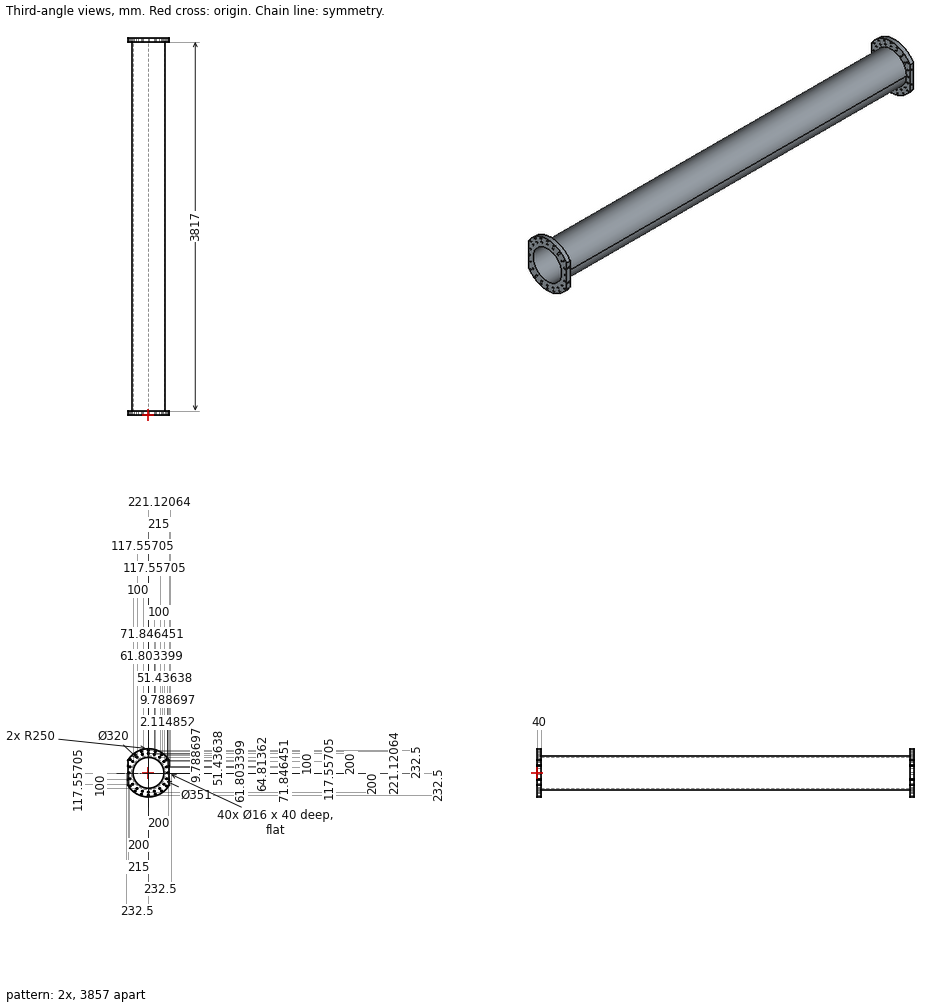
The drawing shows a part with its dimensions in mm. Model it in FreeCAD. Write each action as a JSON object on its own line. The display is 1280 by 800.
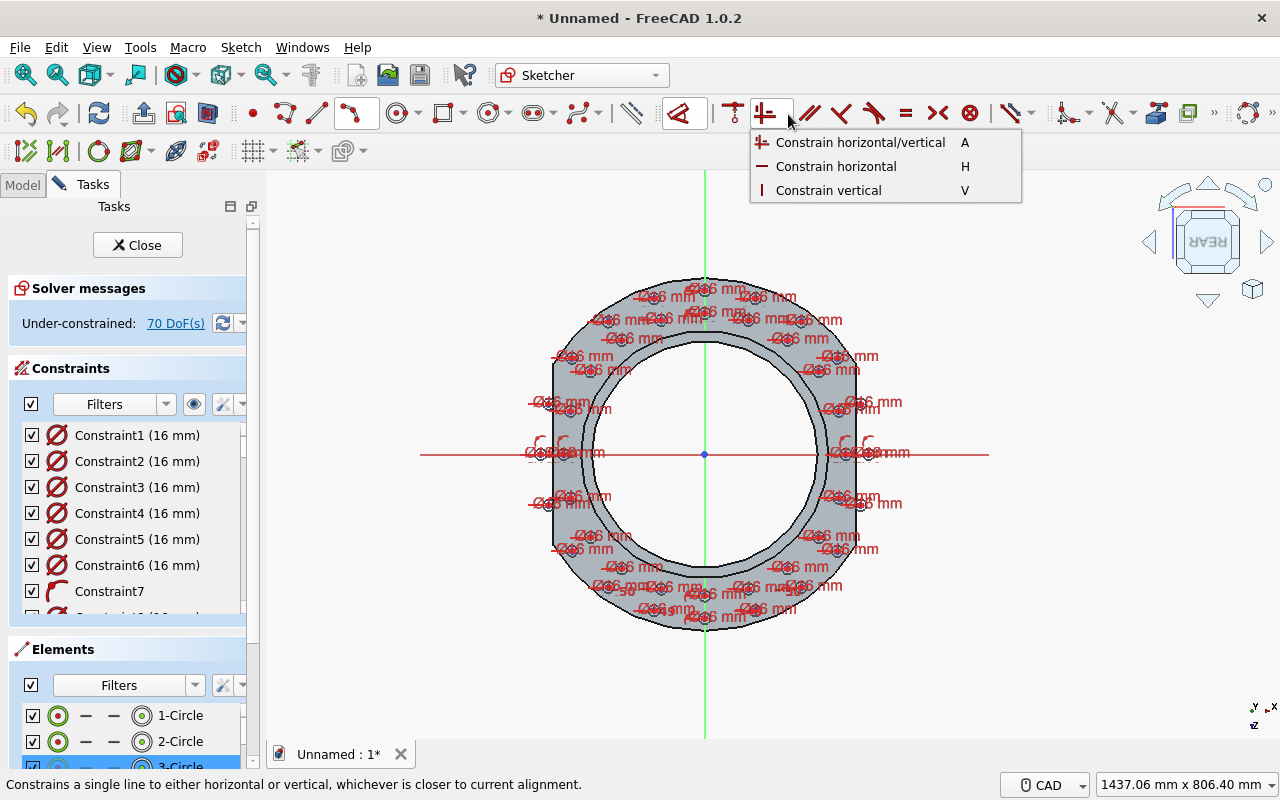
{"action": "left_click", "coordinate": [886, 166]}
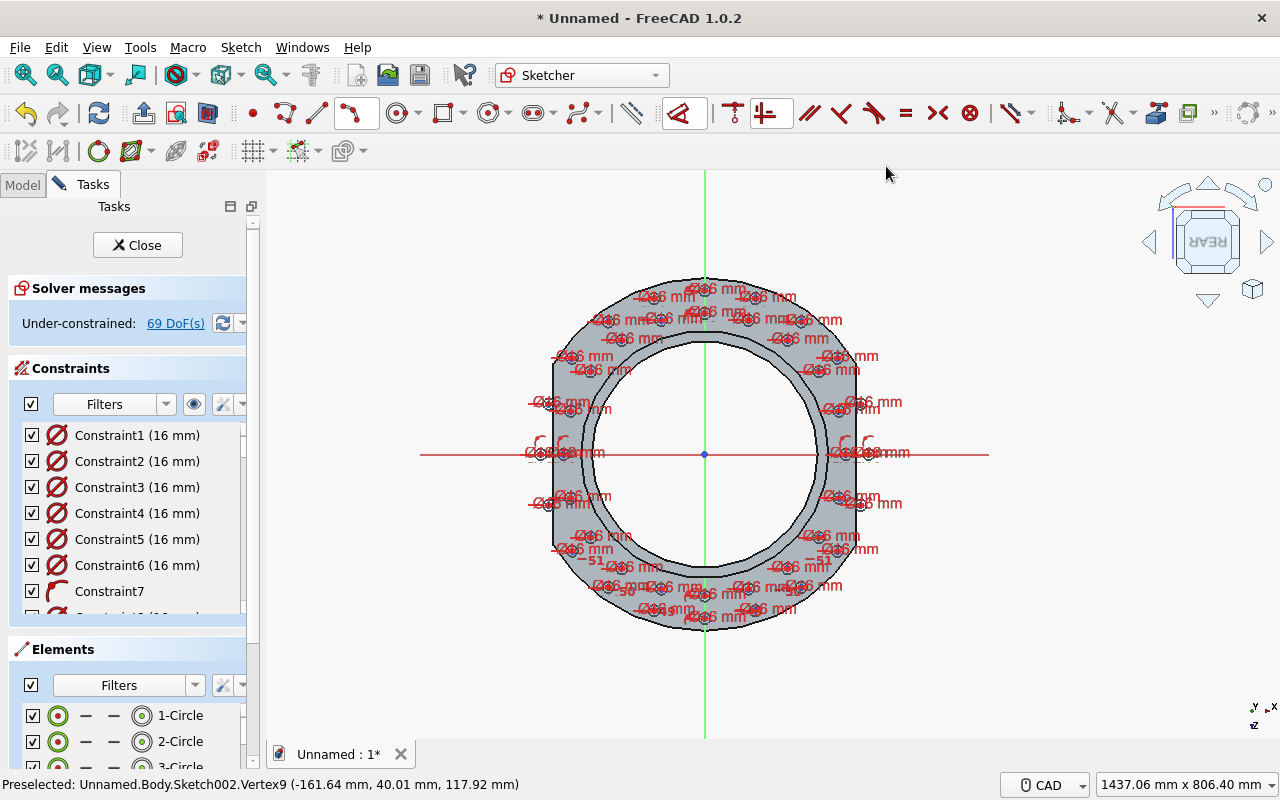
{"action": "left_click", "coordinate": [570, 498]}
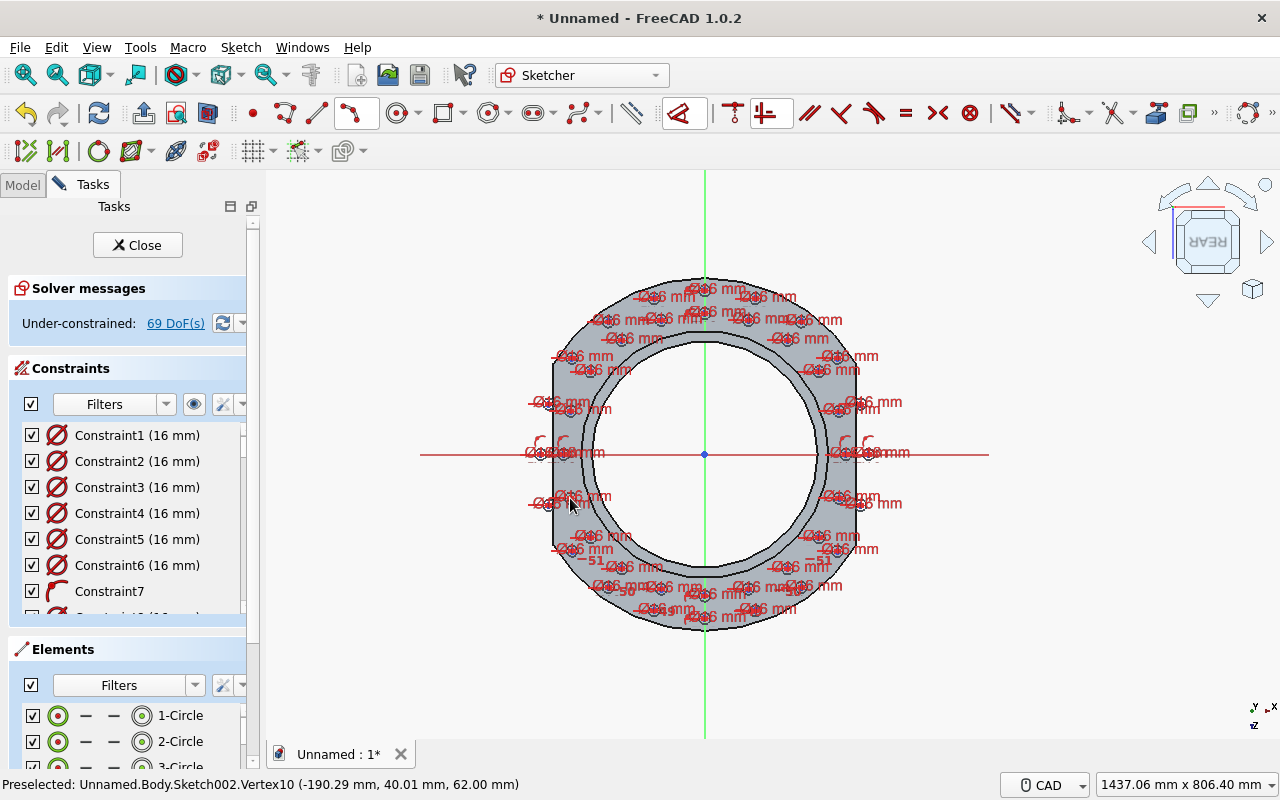
{"action": "left_click", "coordinate": [571, 411]}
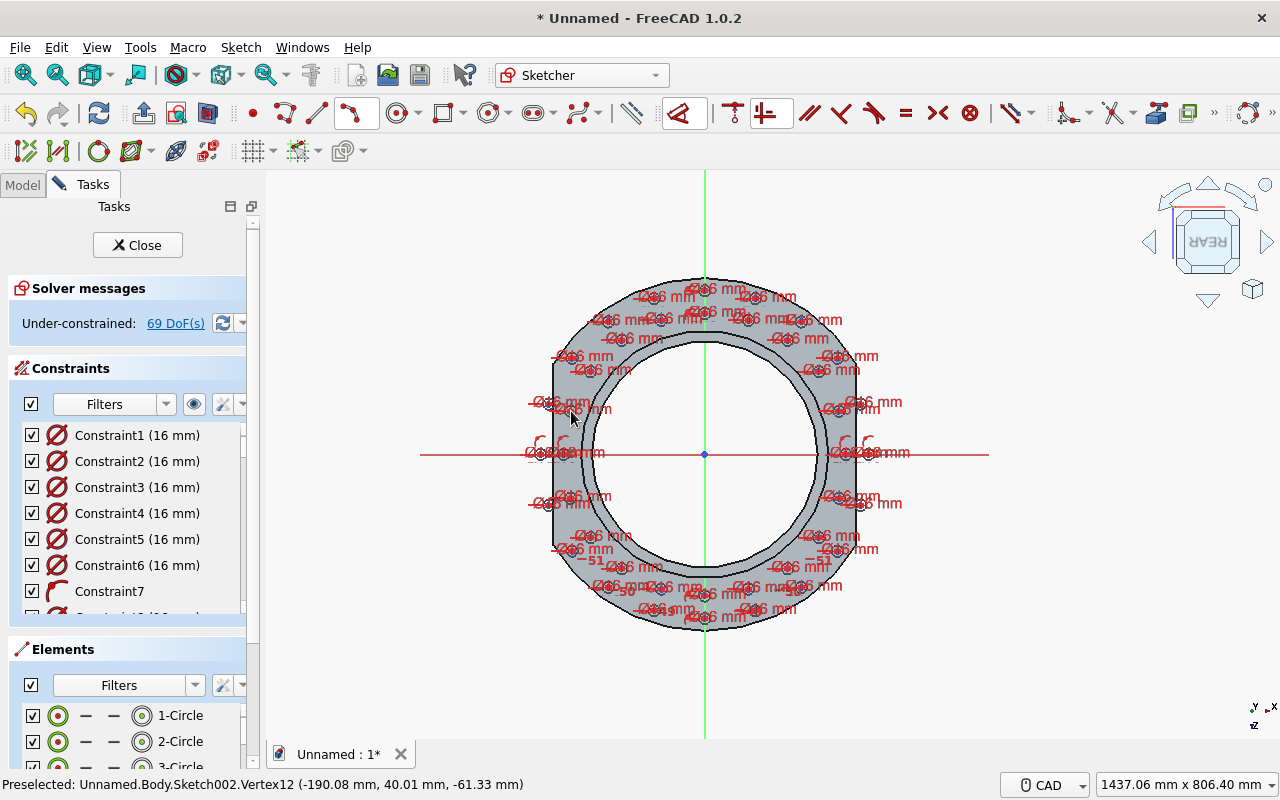
{"action": "left_click", "coordinate": [788, 114]}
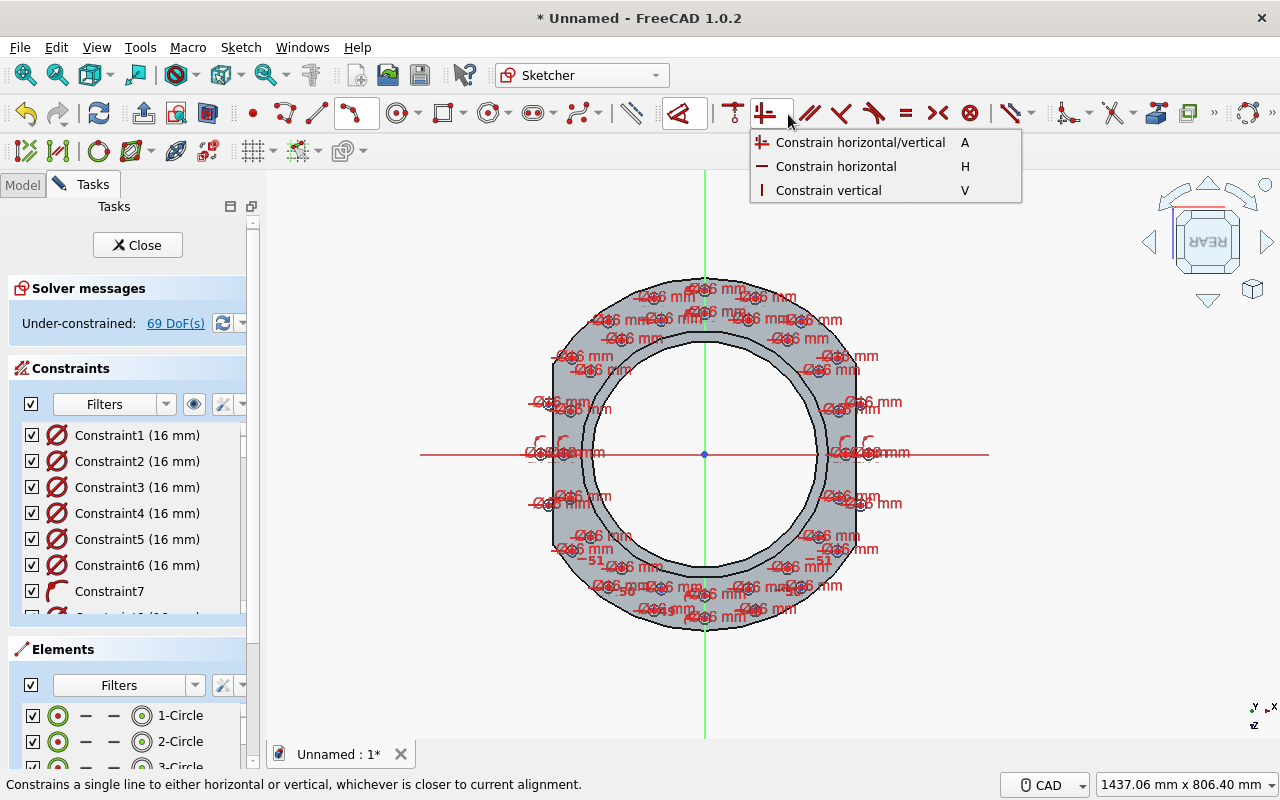
{"action": "left_click", "coordinate": [886, 190]}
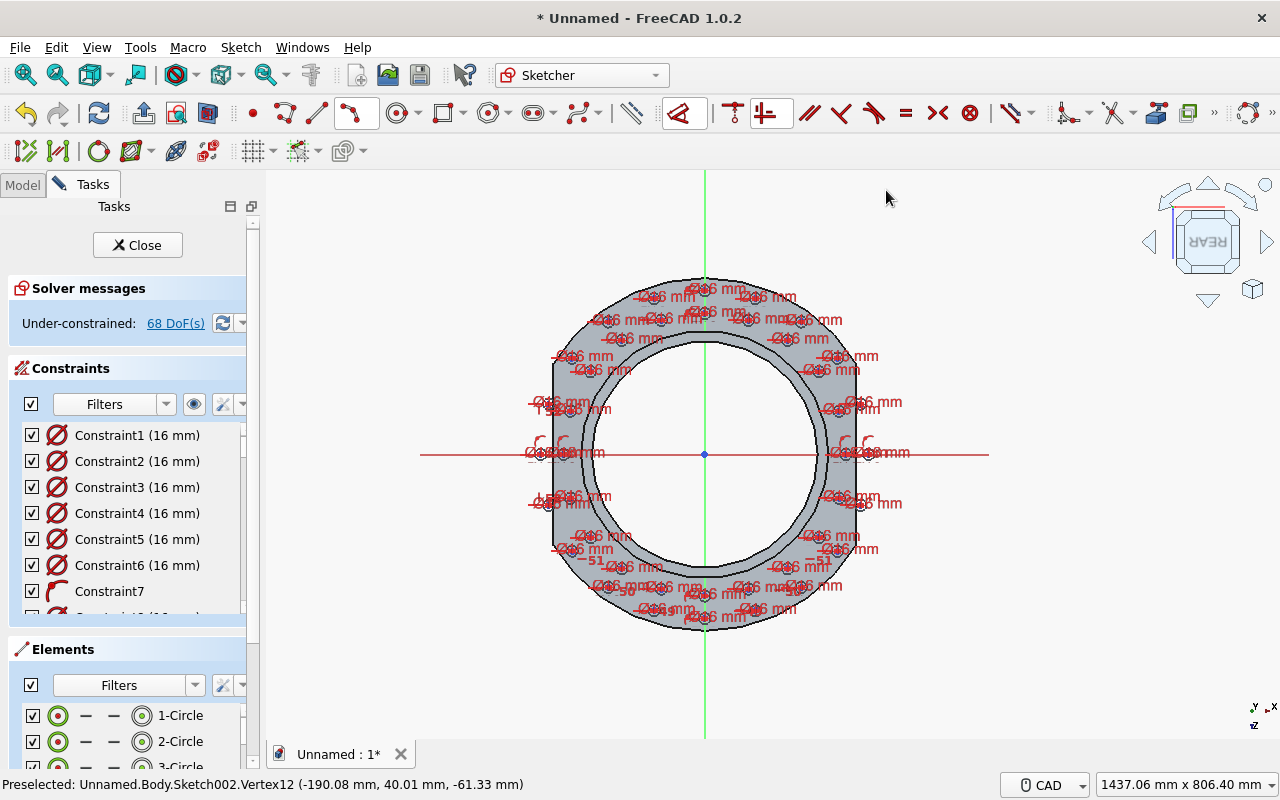
{"action": "left_click", "coordinate": [591, 538]}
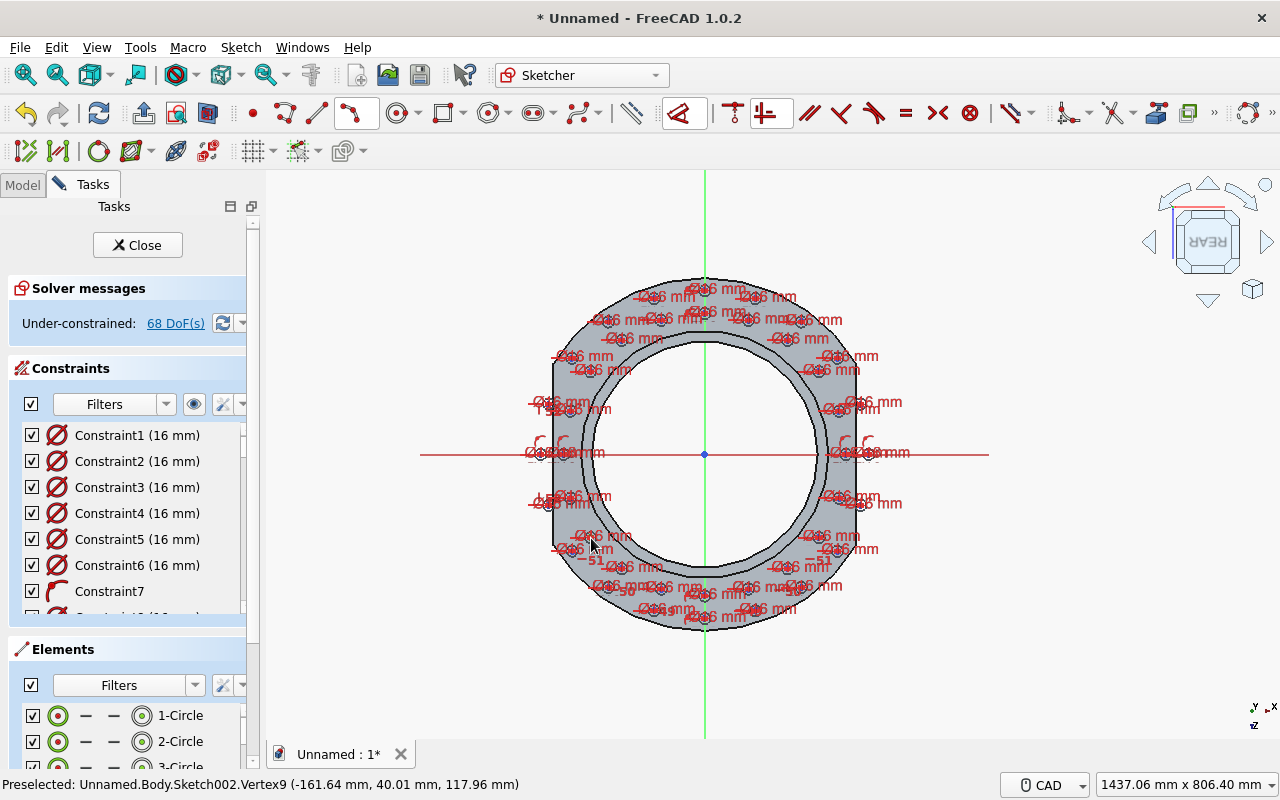
{"action": "left_click", "coordinate": [591, 372]}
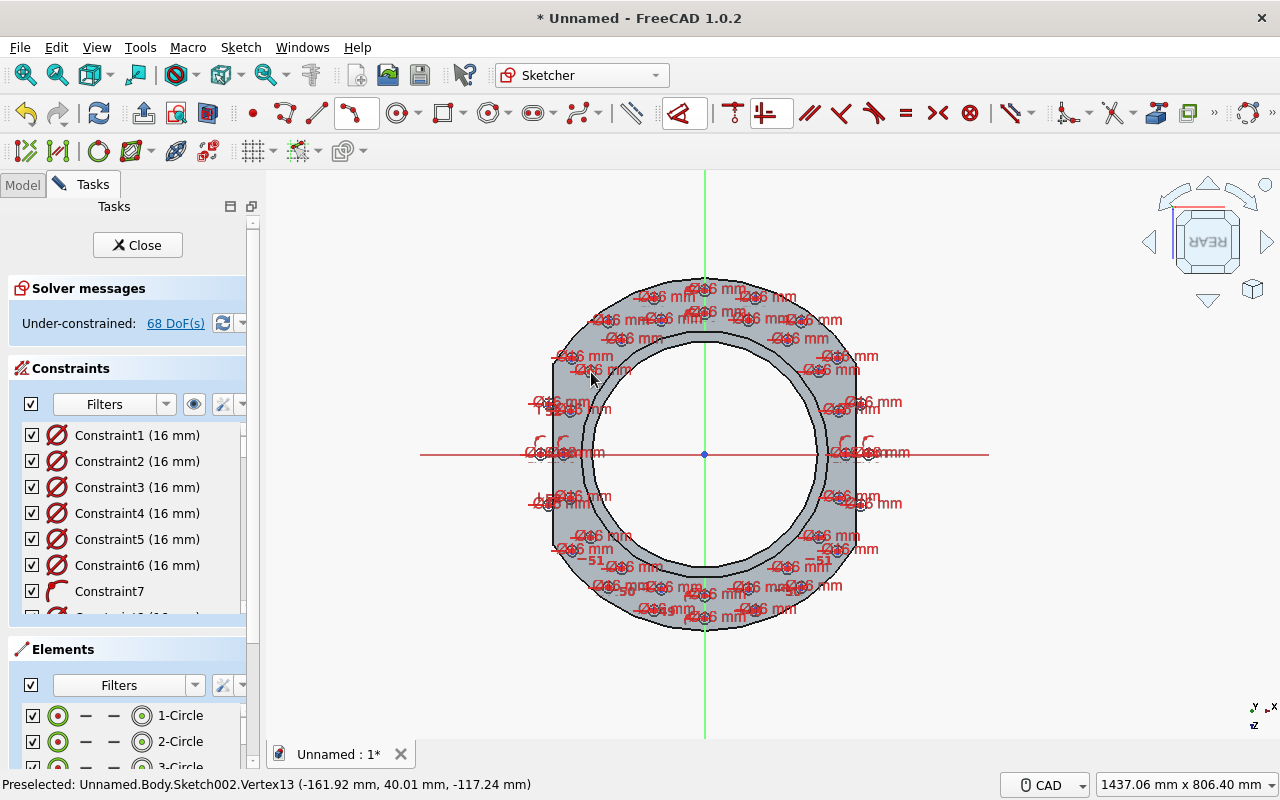
{"action": "key", "text": "v"}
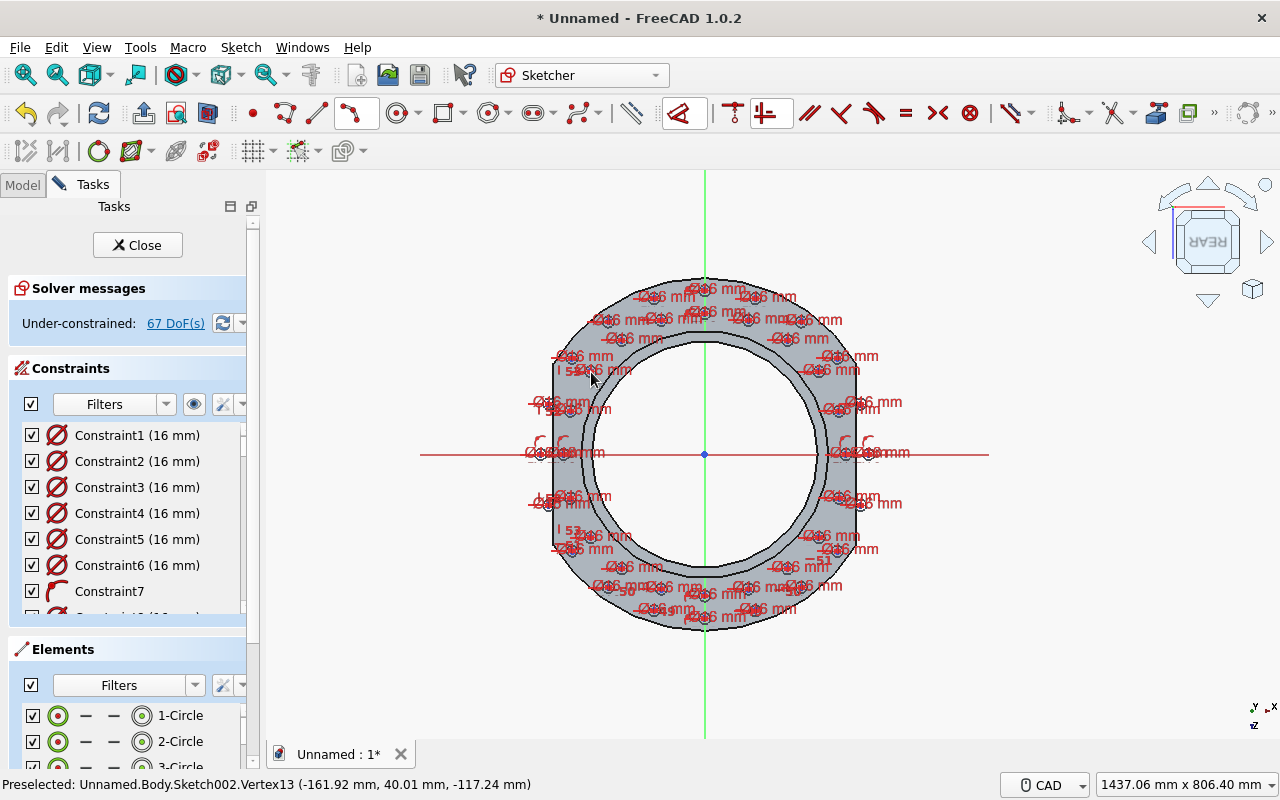
{"action": "left_click", "coordinate": [622, 569]}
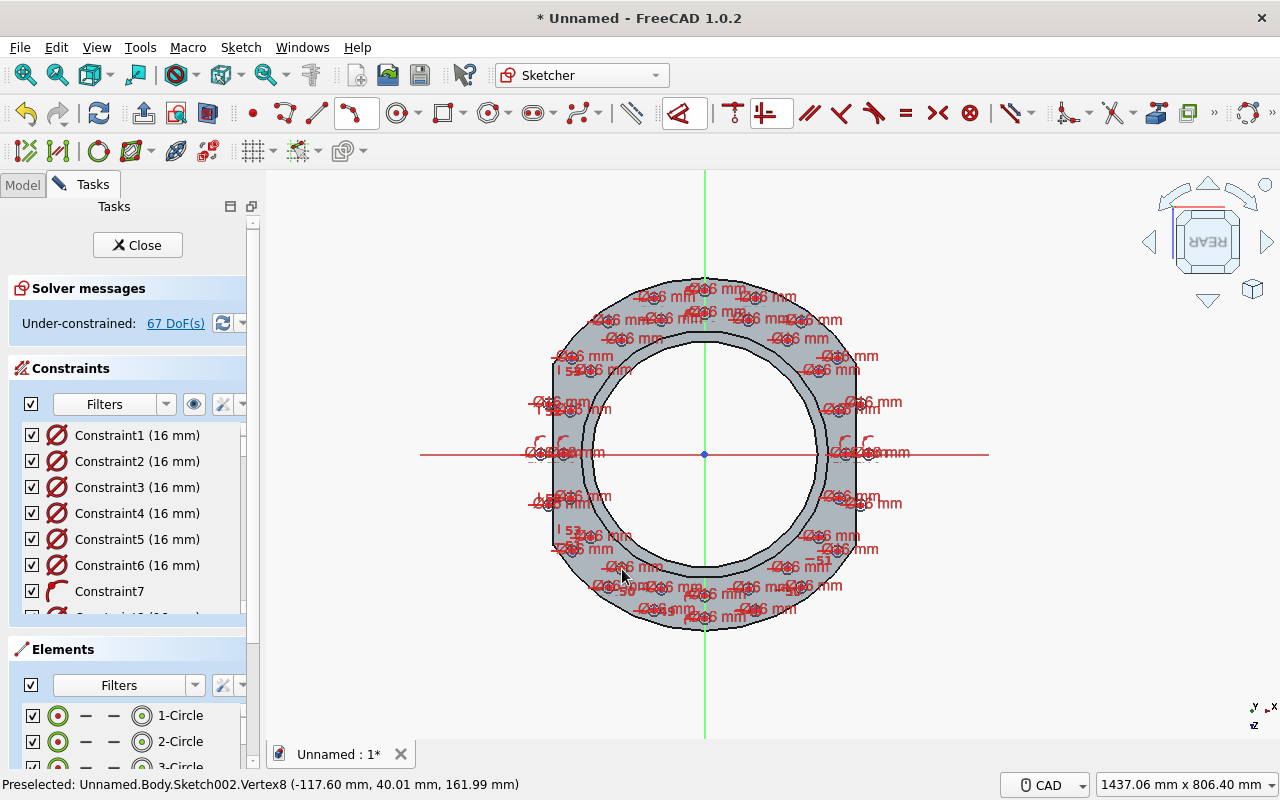
{"action": "left_click", "coordinate": [622, 340]}